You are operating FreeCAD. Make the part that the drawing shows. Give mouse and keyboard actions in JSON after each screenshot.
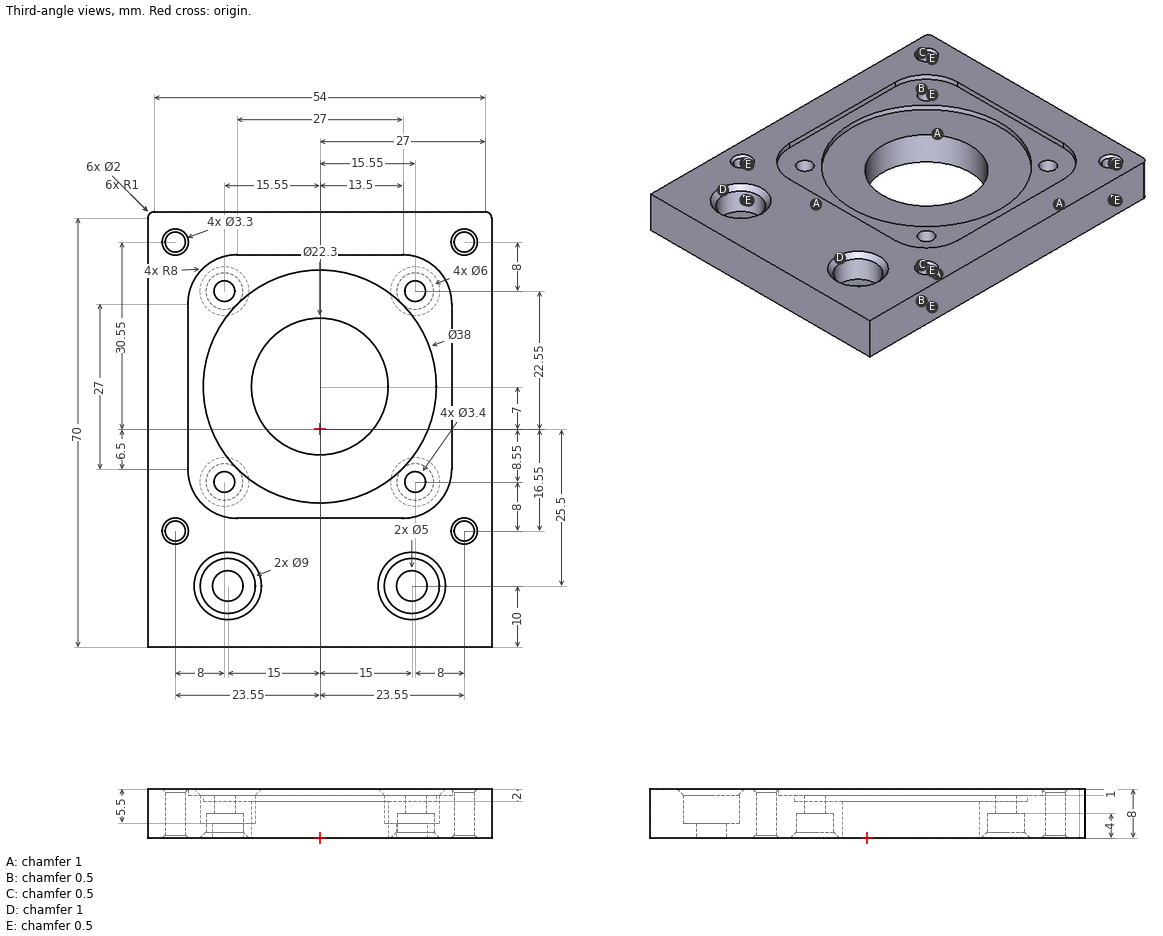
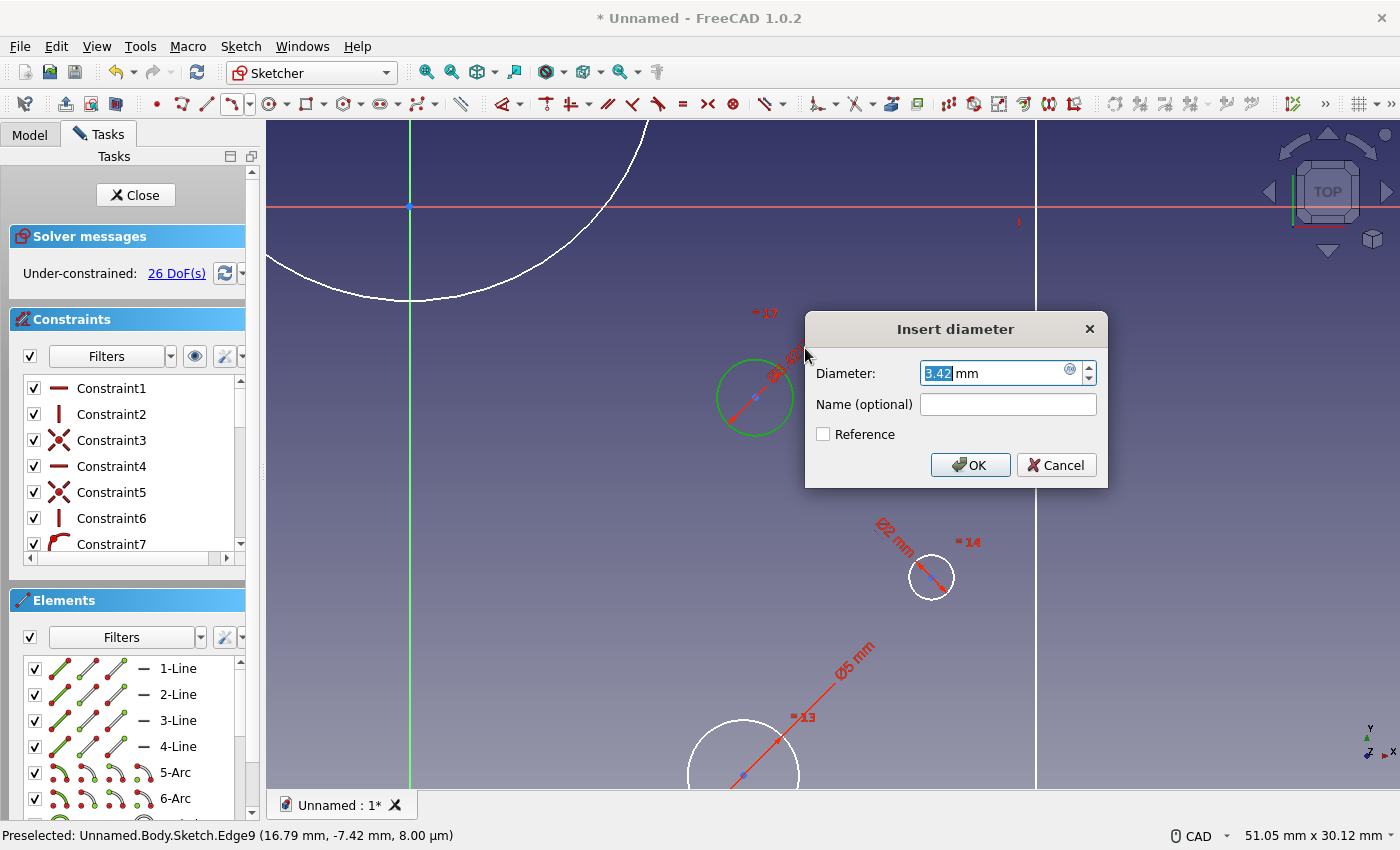
{"action": "type", "text": "3.4"}
{"action": "key", "text": "Return"}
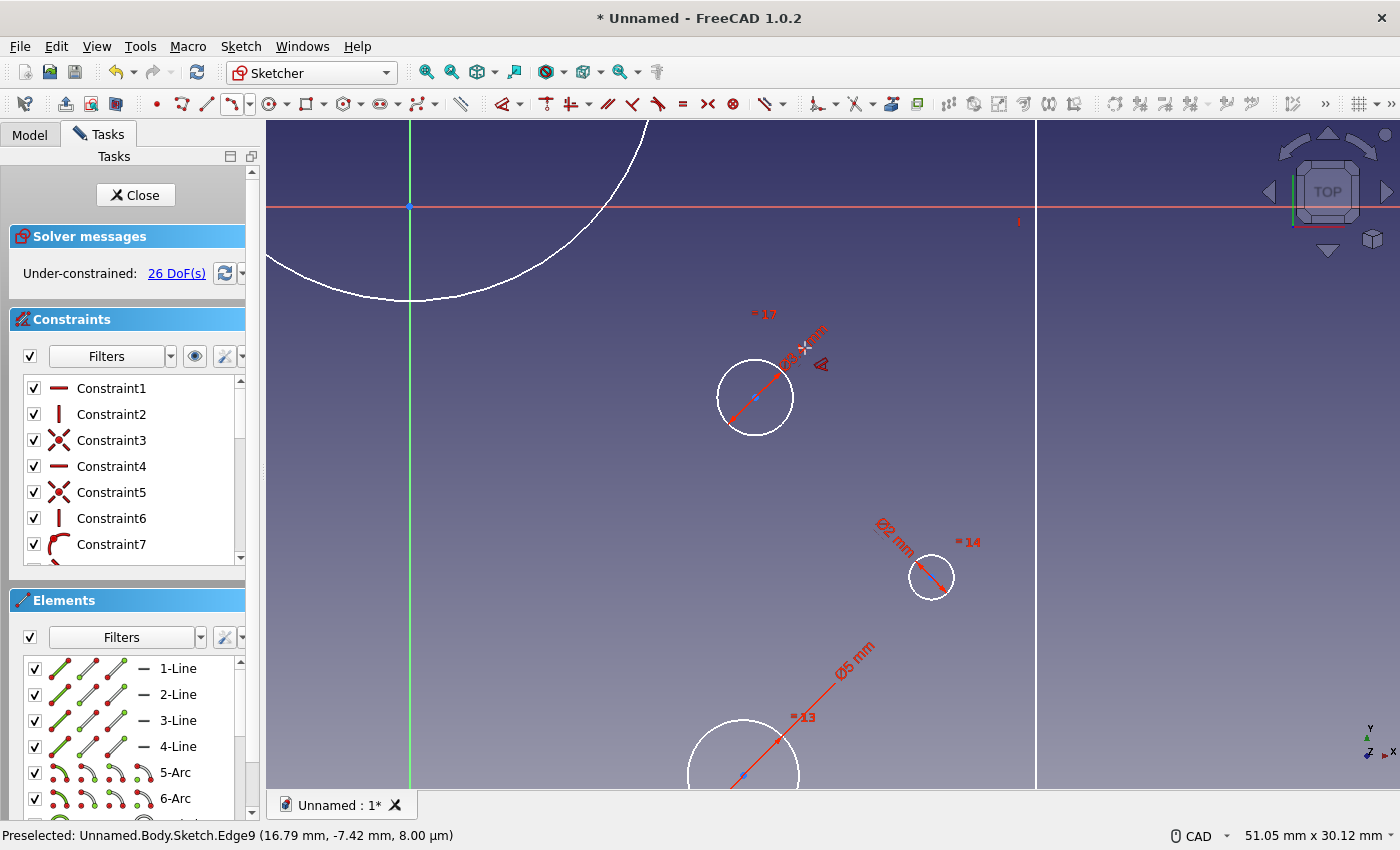
{"action": "left_click", "coordinate": [586, 228]}
{"action": "left_click", "coordinate": [609, 251]}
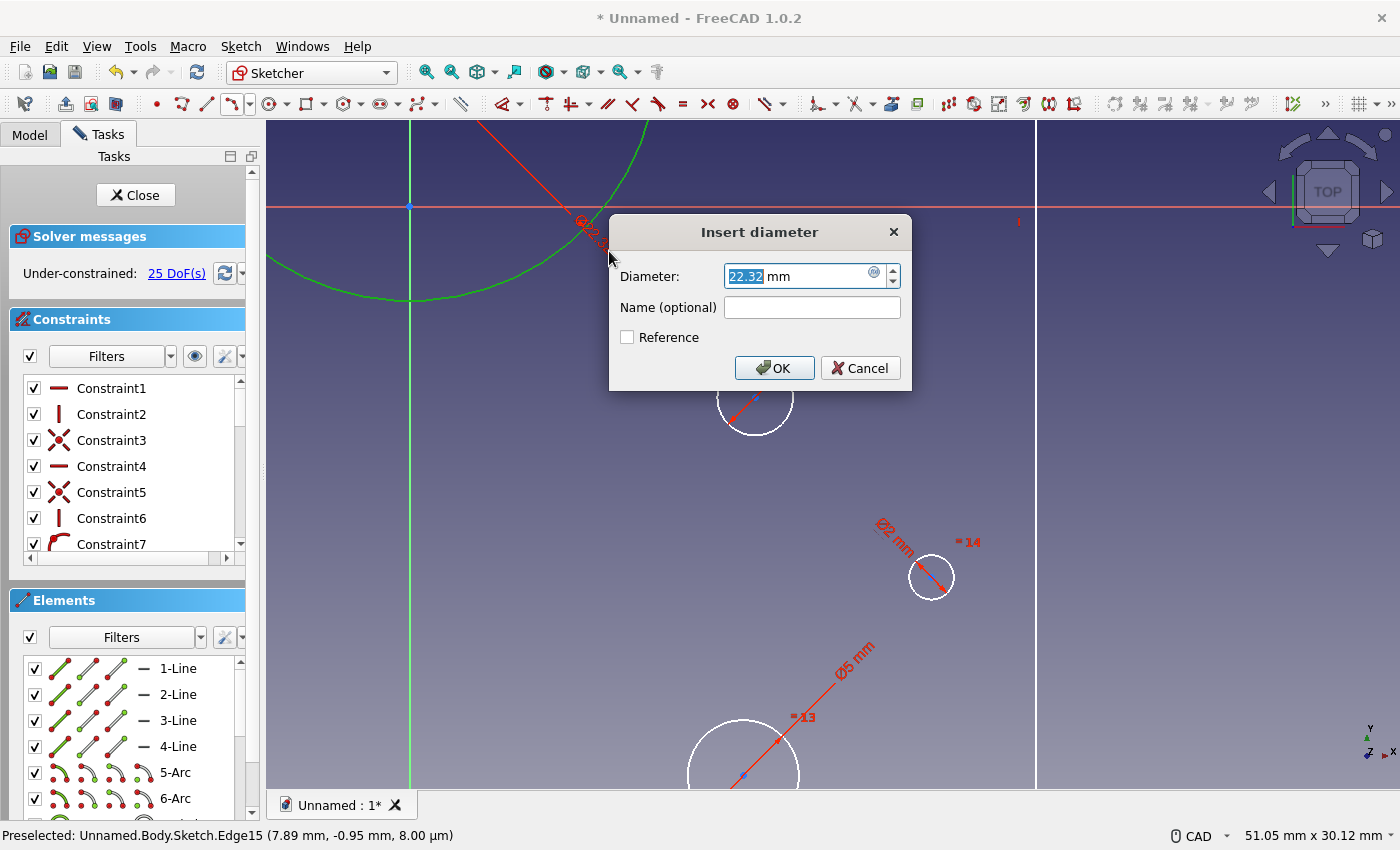
{"action": "type", "text": "22.3"}
{"action": "key", "text": "Return"}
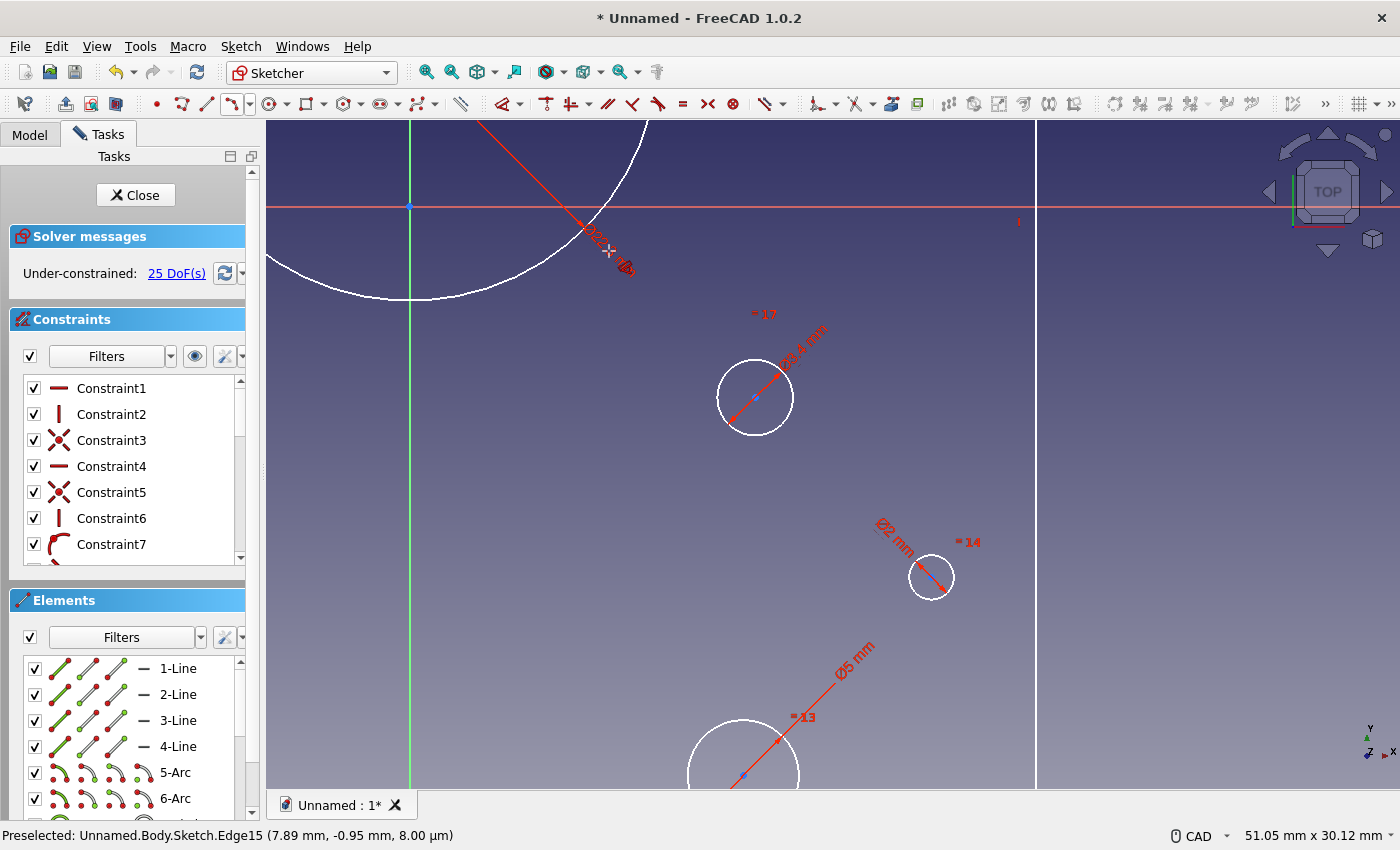
{"action": "scroll", "coordinate": [917, 561], "scroll_direction": "down", "scroll_amount": 6}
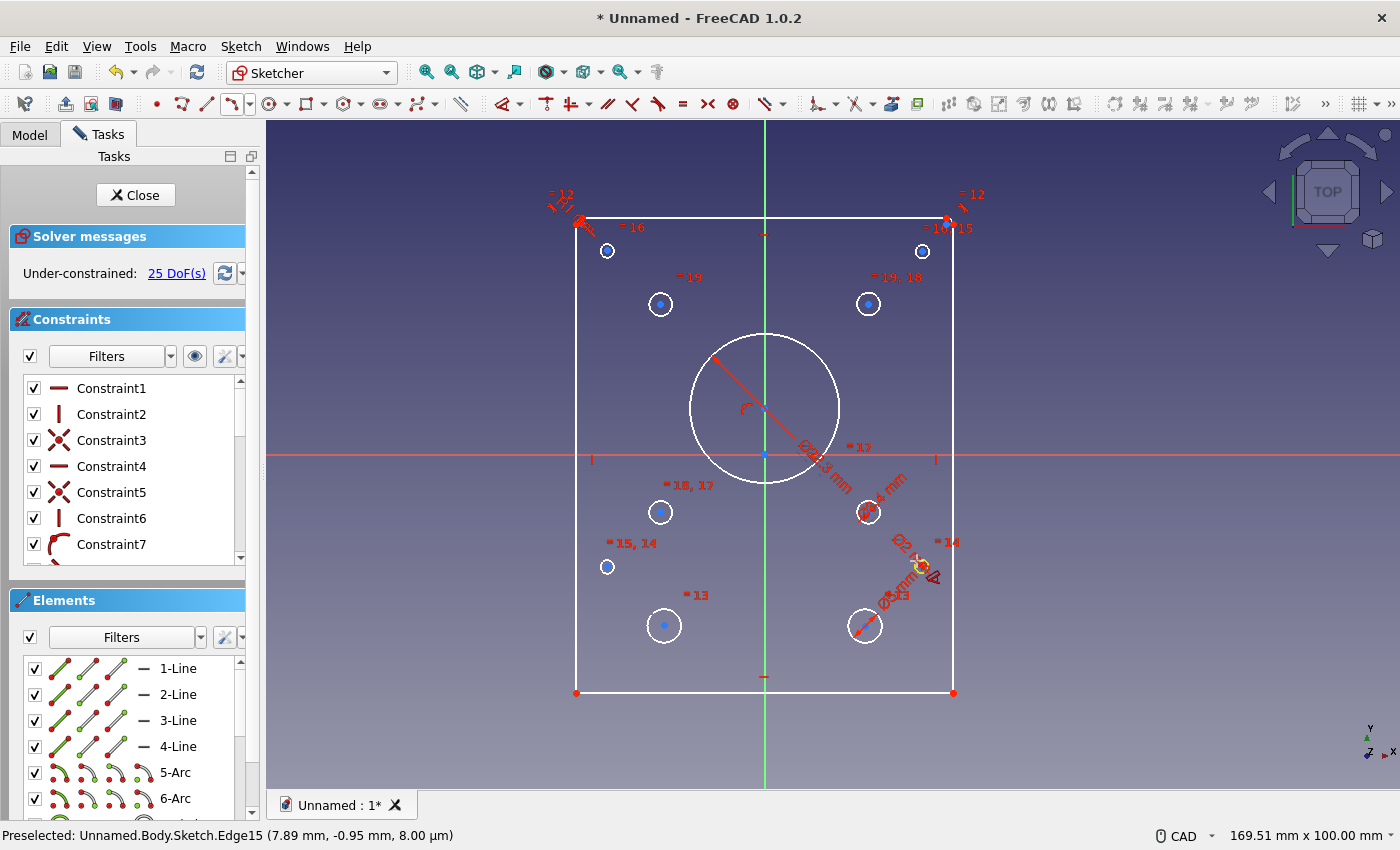
{"action": "left_click", "coordinate": [765, 408]}
{"action": "left_click", "coordinate": [799, 432]}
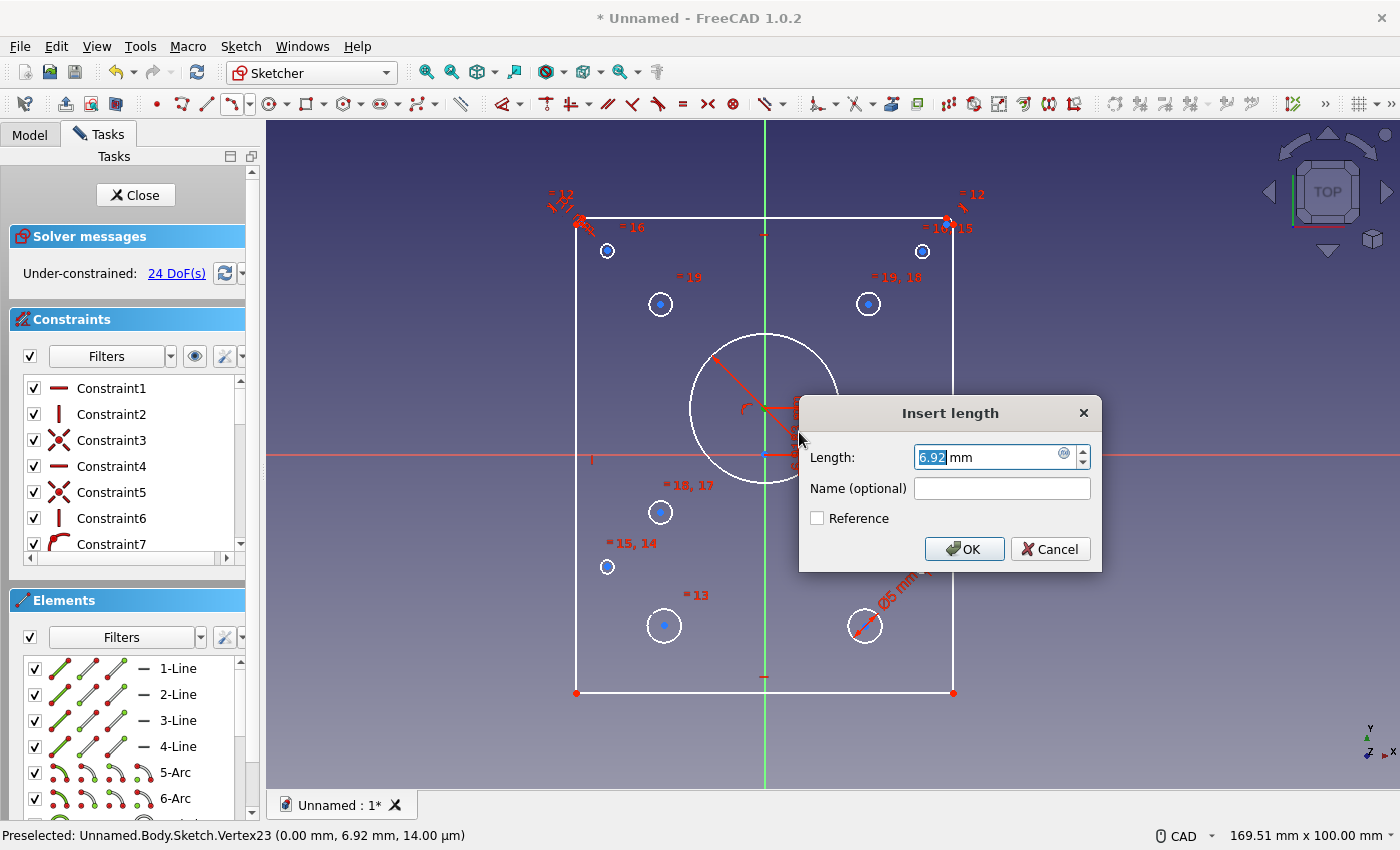
{"action": "type", "text": "7"}
{"action": "key", "text": "Return"}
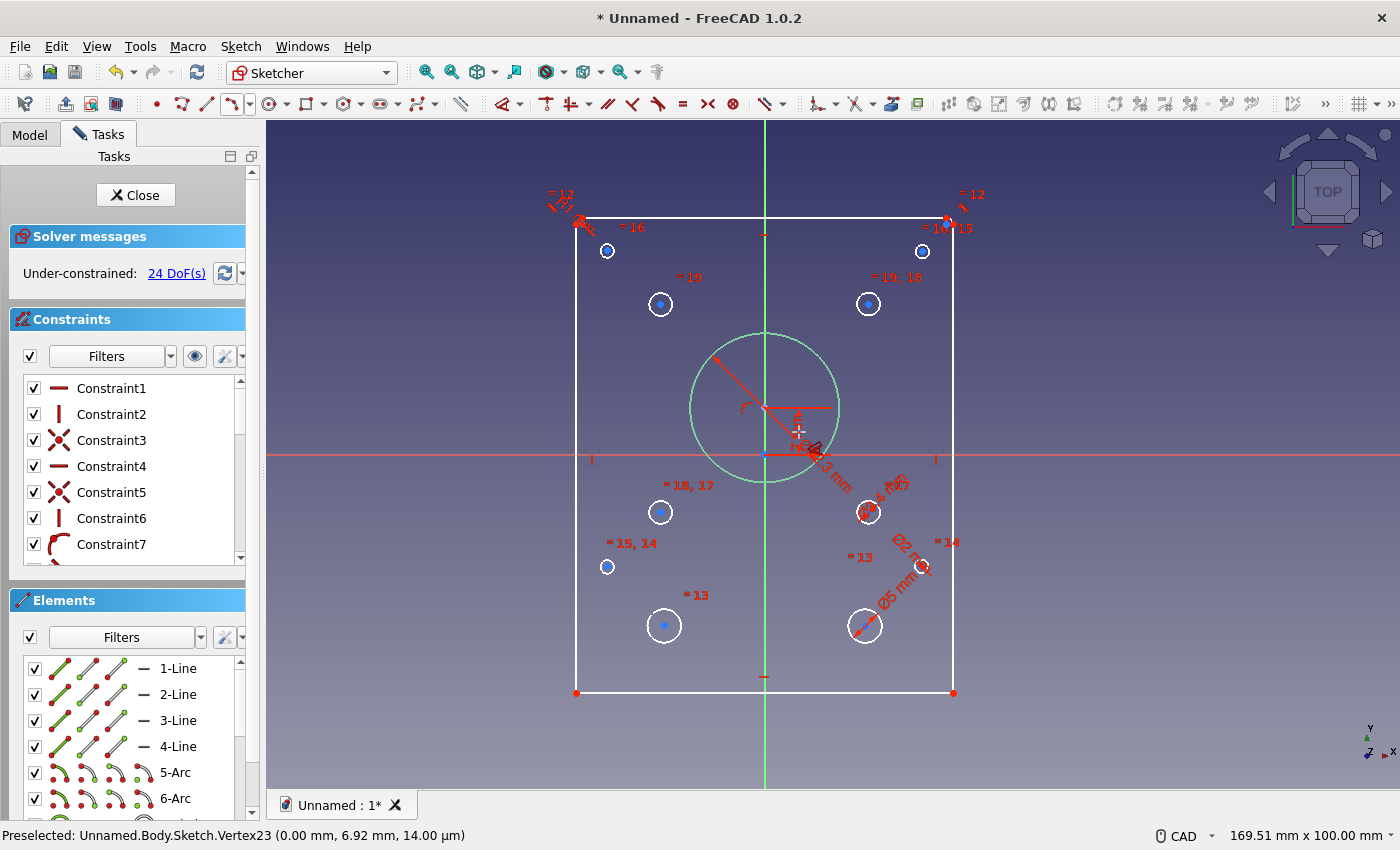
{"action": "left_click", "coordinate": [838, 218]}
{"action": "left_click", "coordinate": [681, 184]}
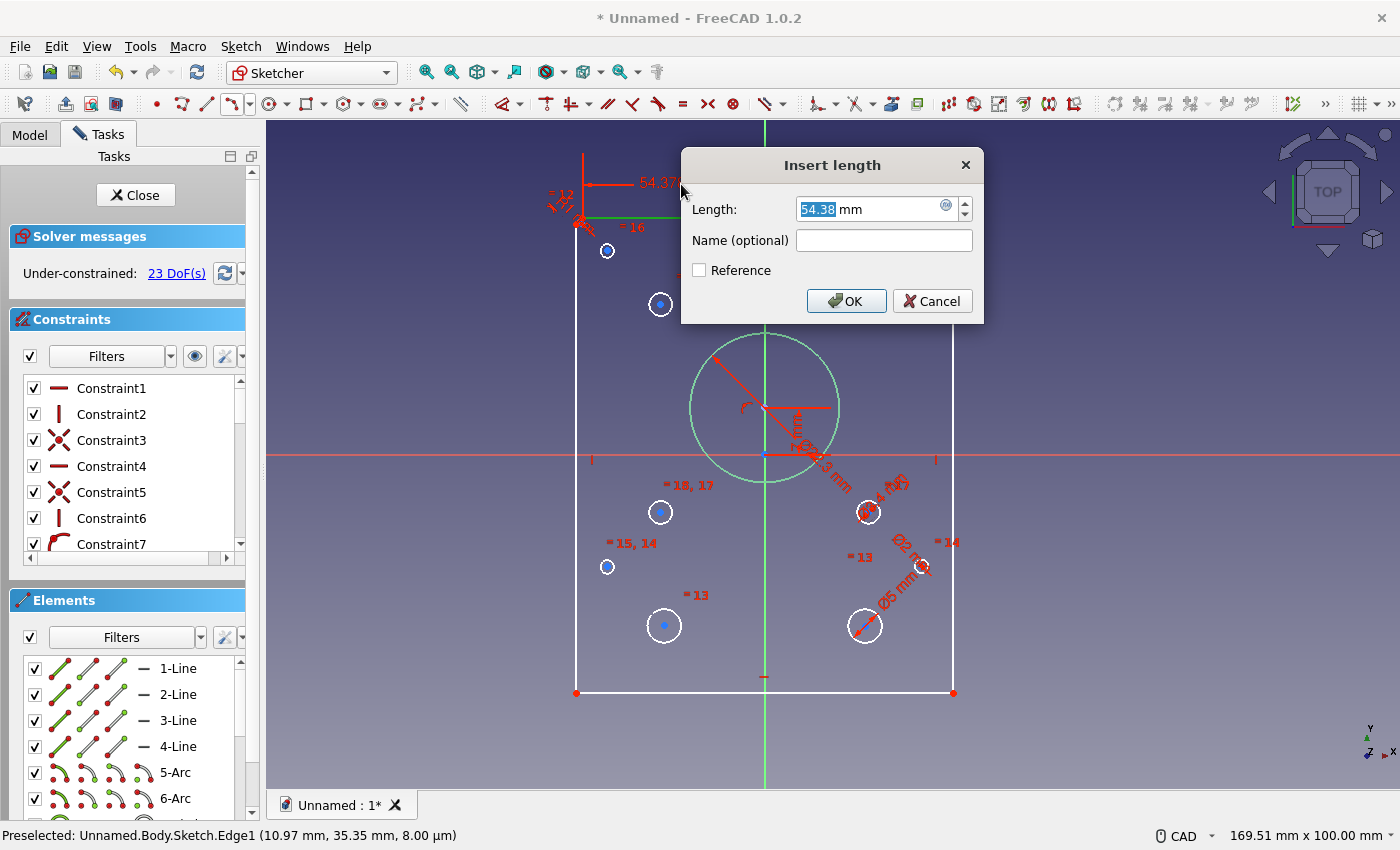
{"action": "type", "text": "54"}
{"action": "key", "text": "Return"}